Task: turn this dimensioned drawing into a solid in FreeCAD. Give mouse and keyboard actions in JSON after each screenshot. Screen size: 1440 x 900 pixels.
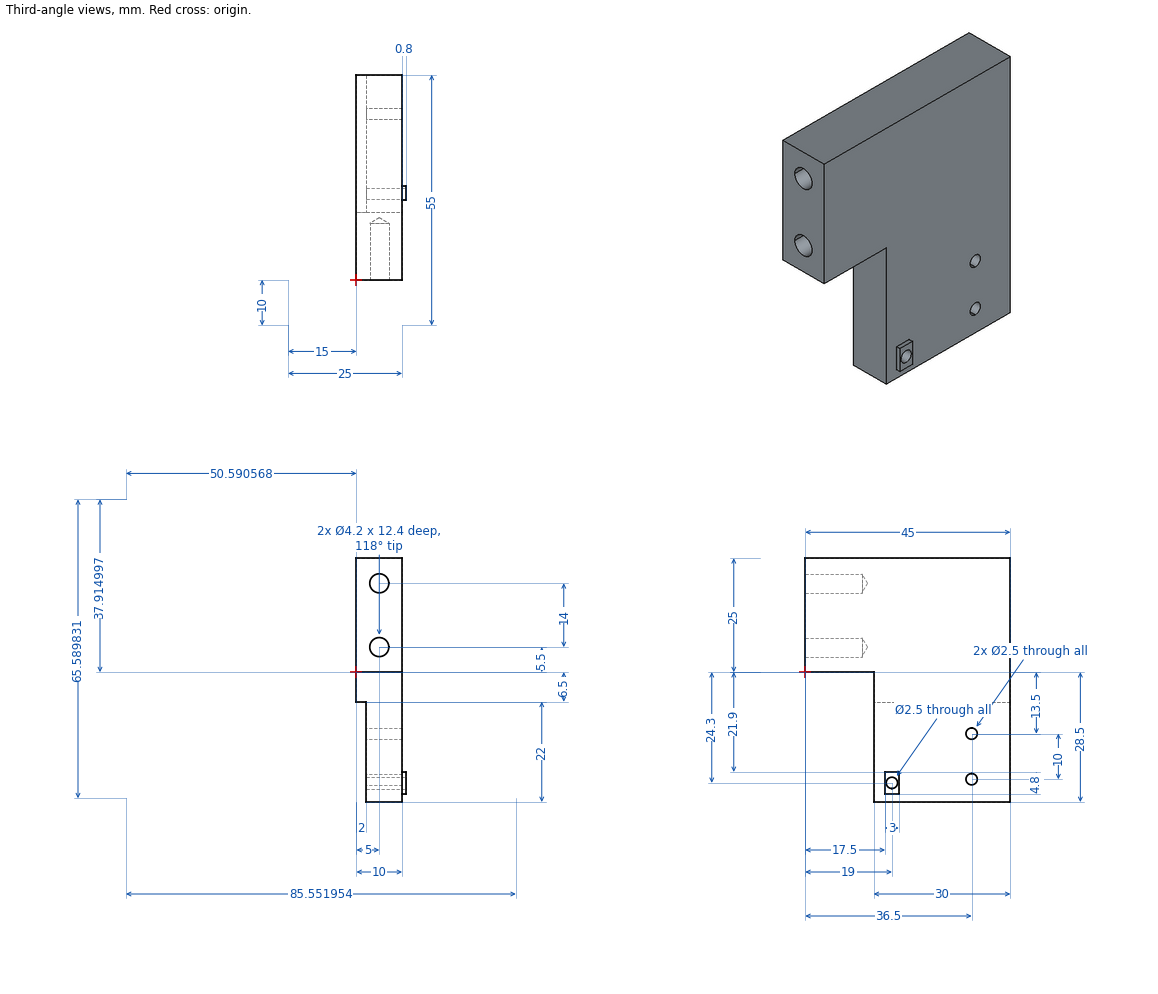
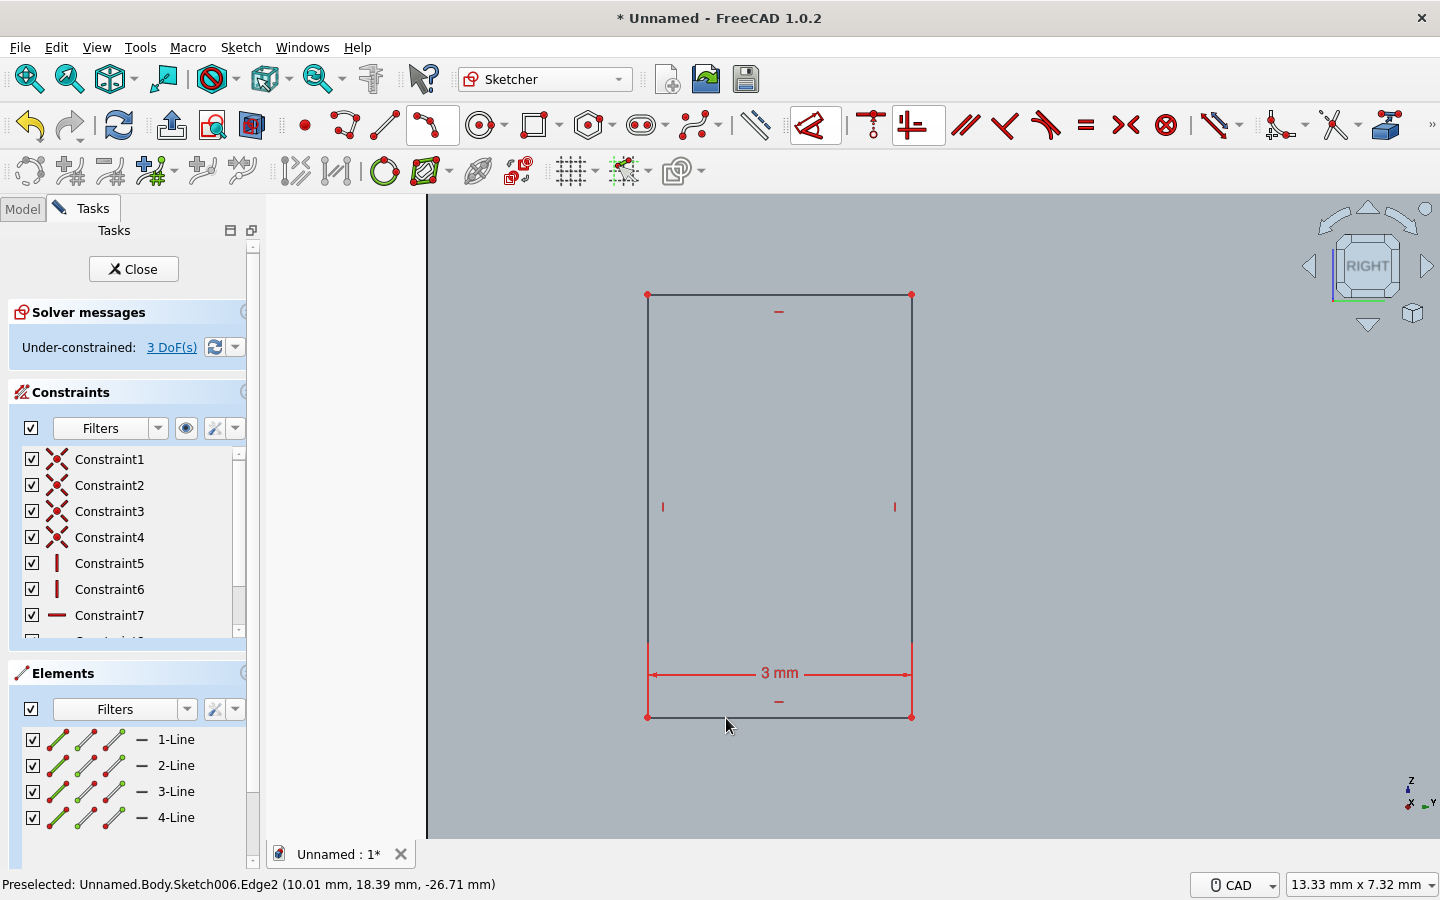
{"action": "left_click", "coordinate": [648, 422]}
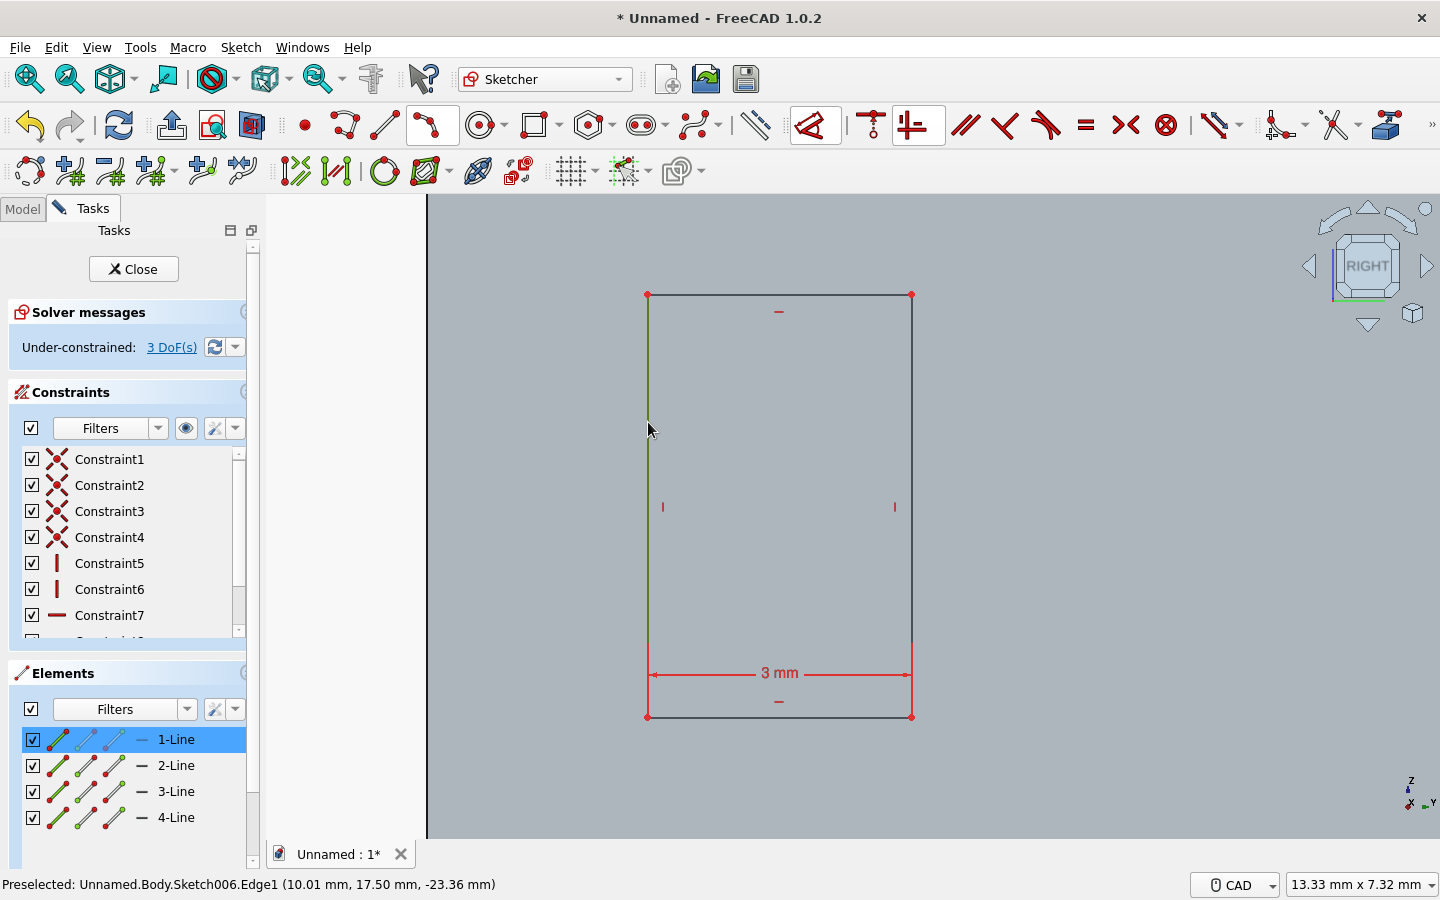
{"action": "key", "text": "i"}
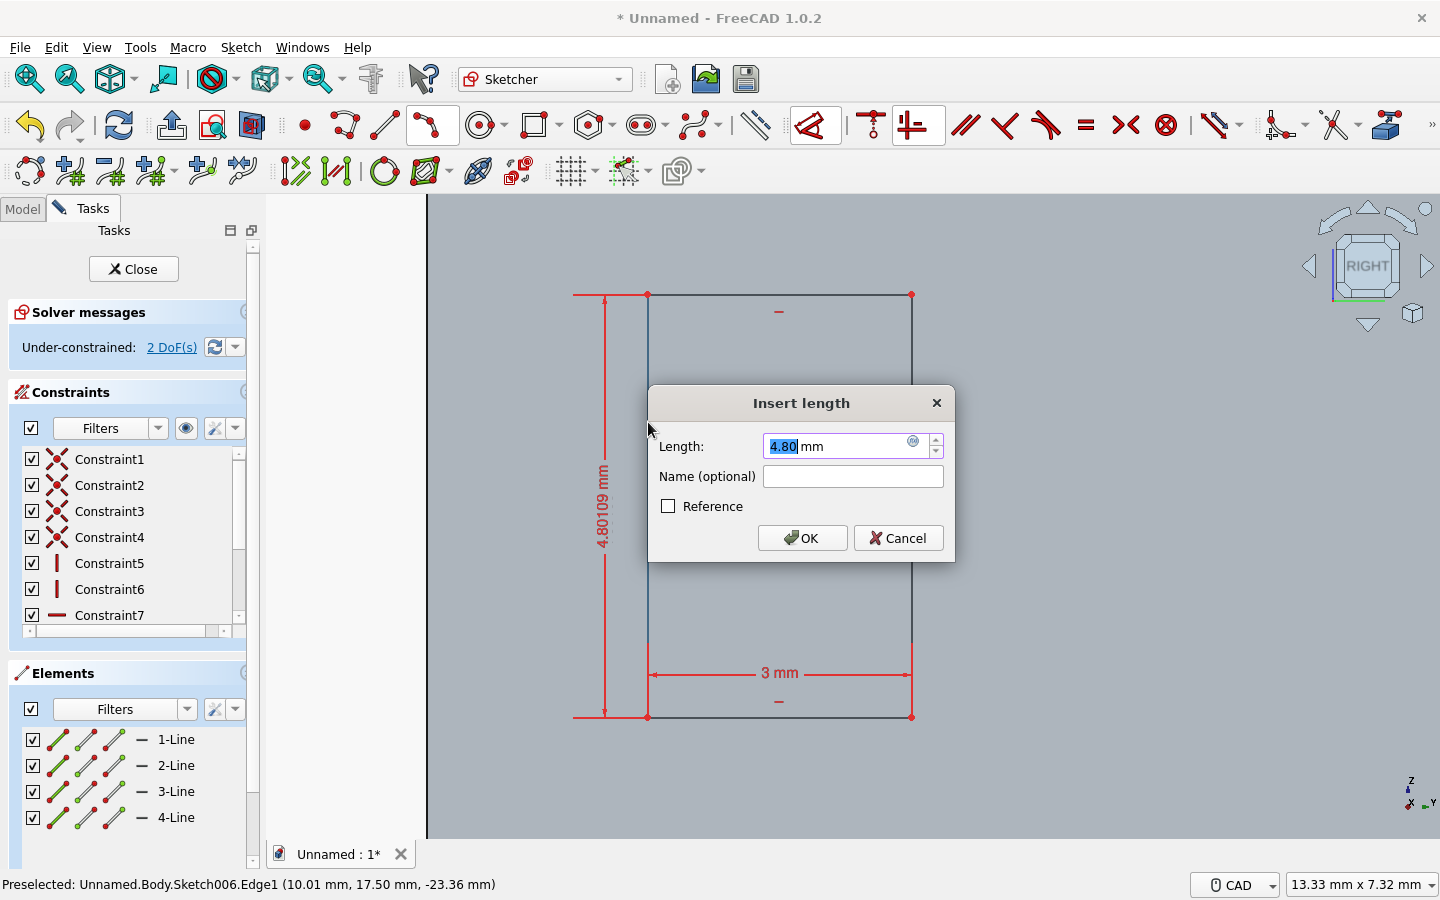
{"action": "type", "text": "4.8"}
{"action": "key", "text": "Return"}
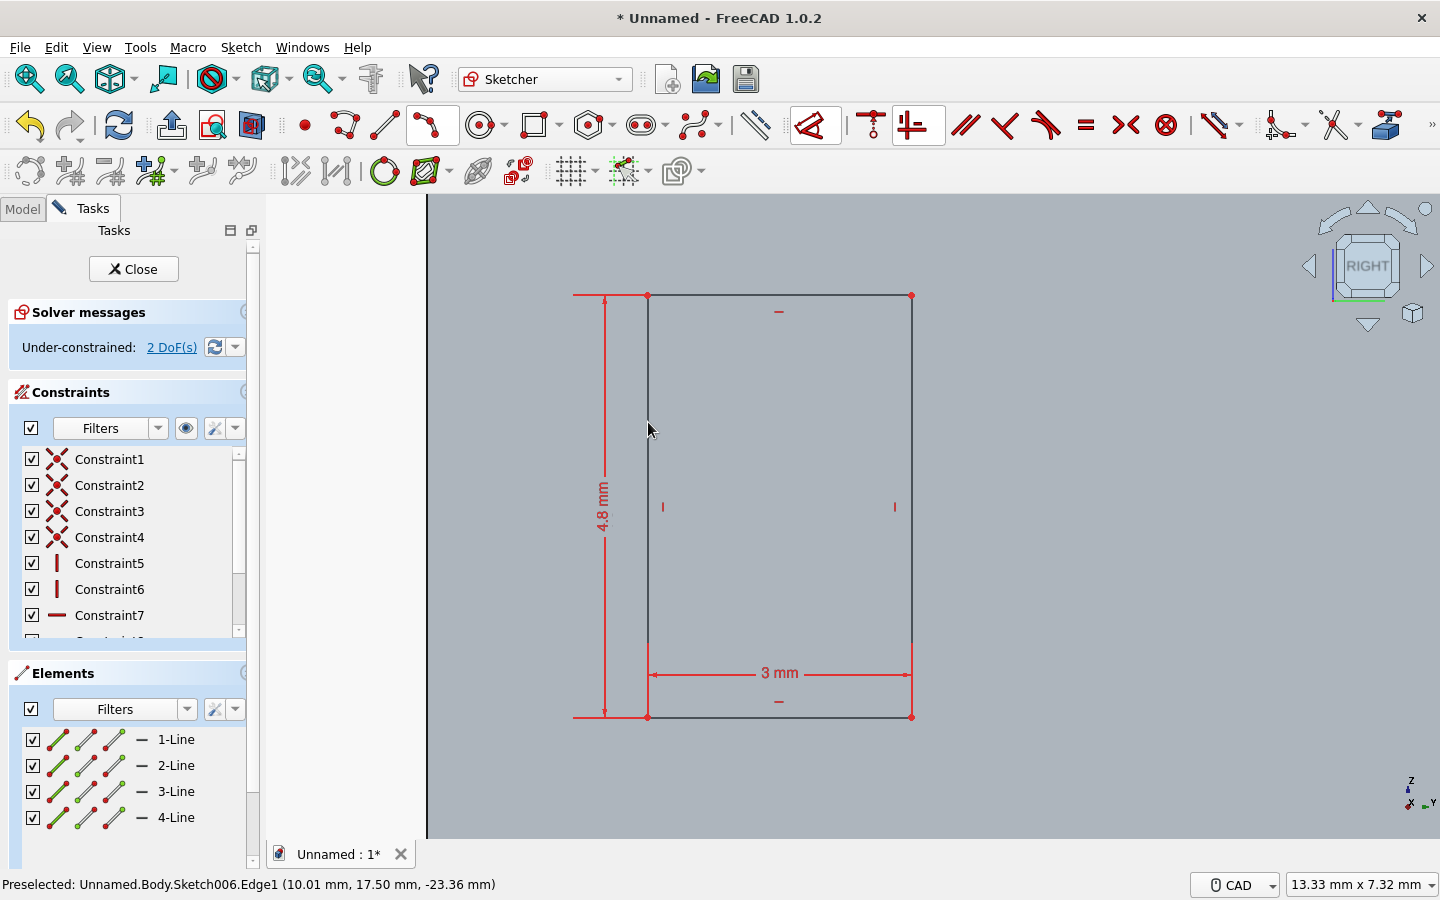
{"action": "left_click", "coordinate": [648, 295]}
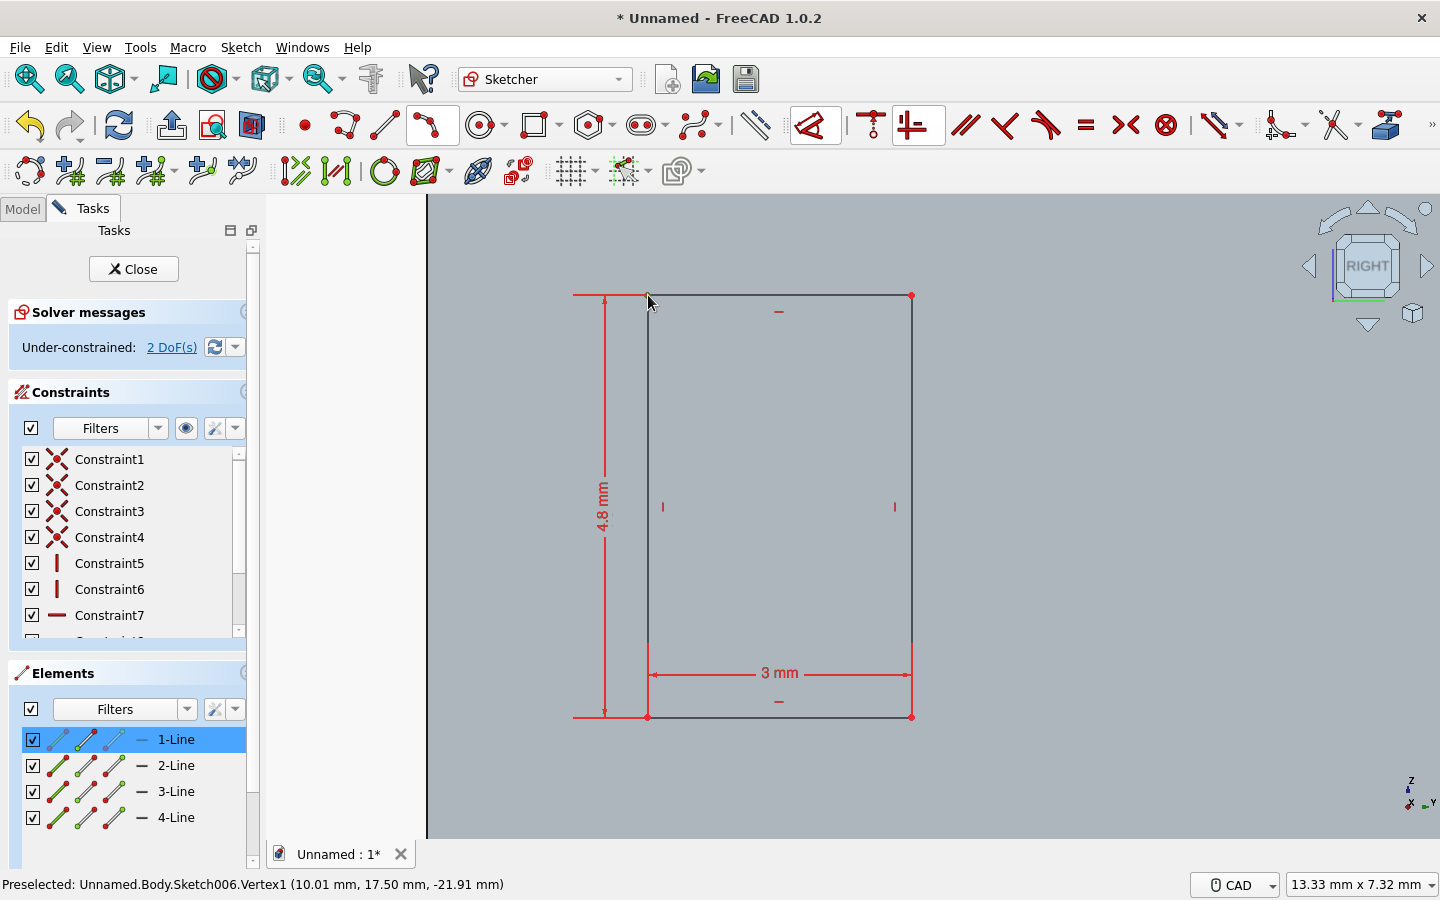
{"action": "left_click", "coordinate": [836, 126]}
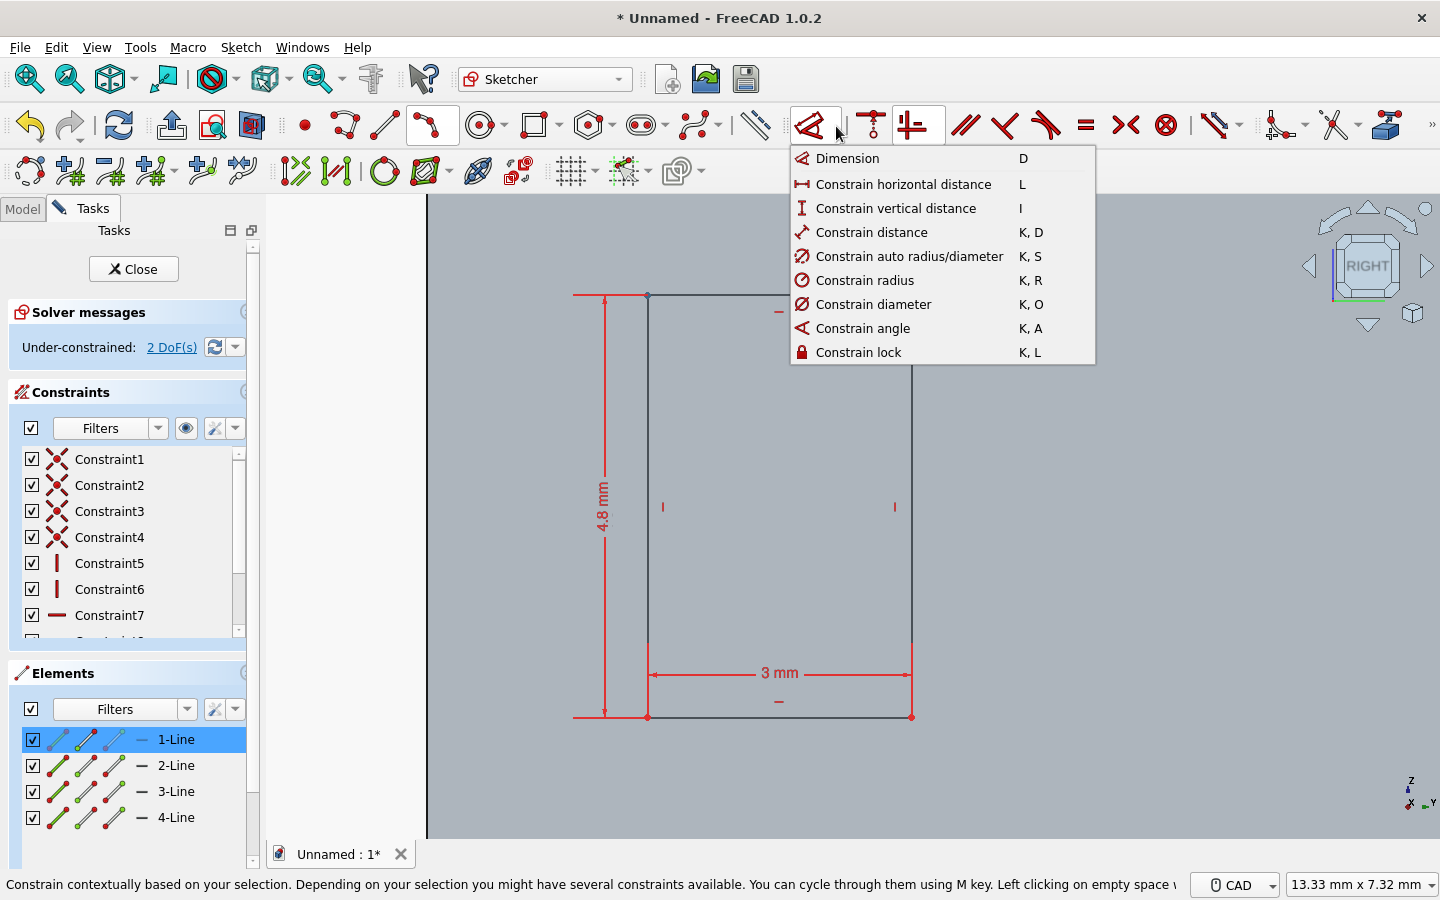
{"action": "left_click", "coordinate": [943, 184]}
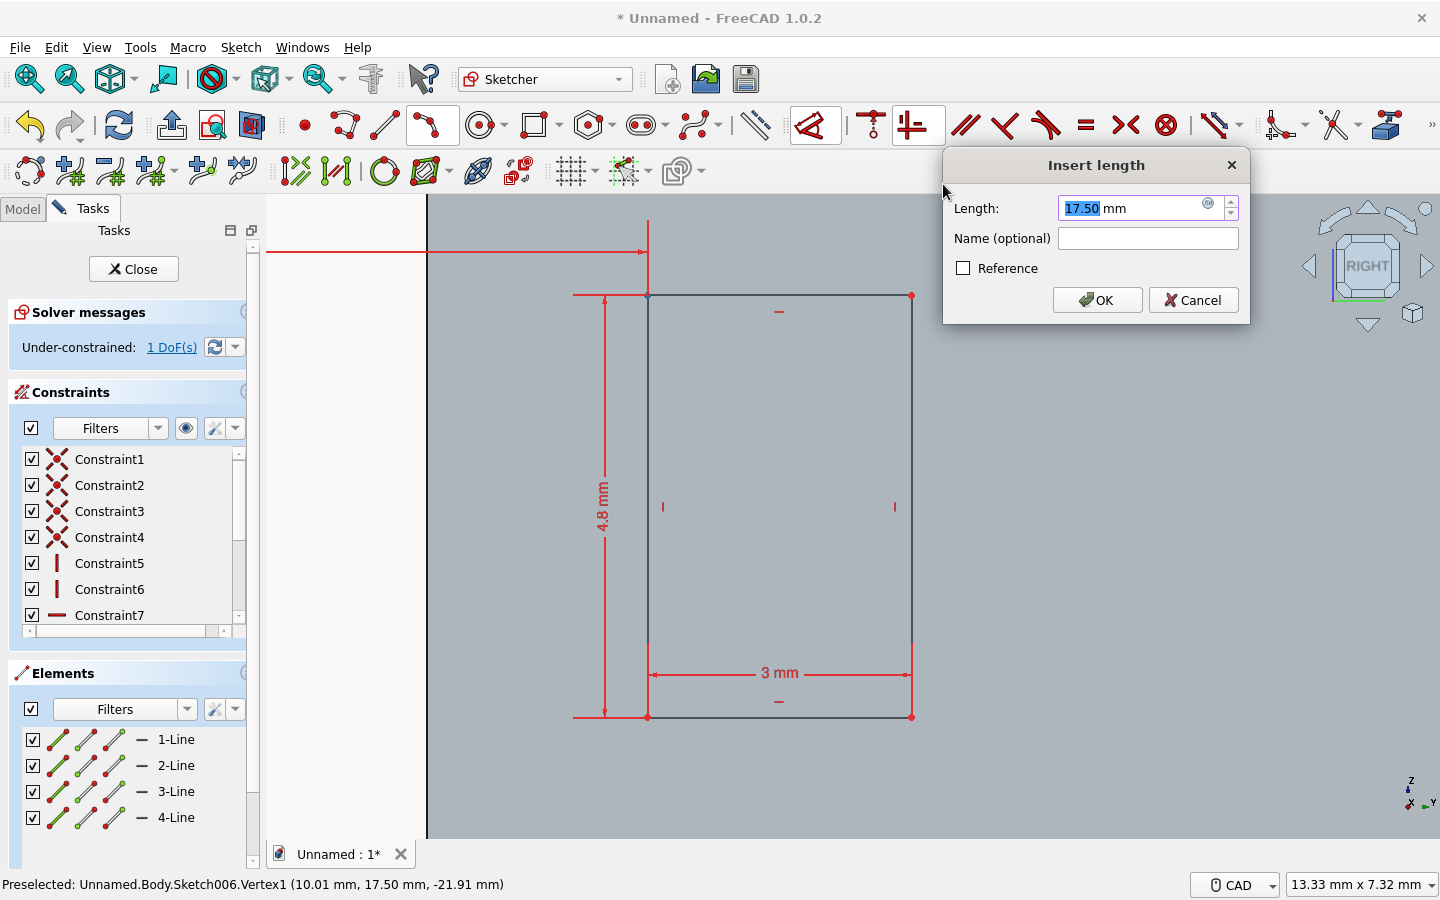
{"action": "type", "text": "17.5"}
{"action": "key", "text": "Return"}